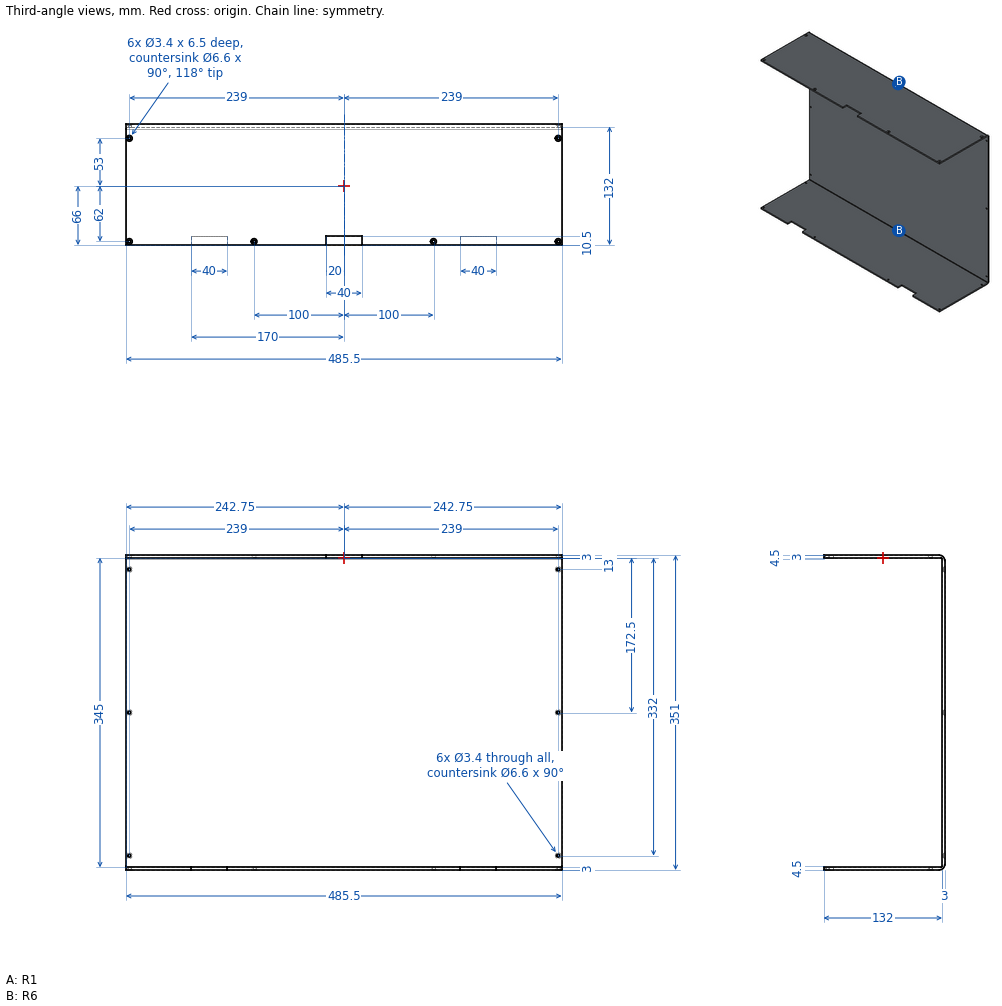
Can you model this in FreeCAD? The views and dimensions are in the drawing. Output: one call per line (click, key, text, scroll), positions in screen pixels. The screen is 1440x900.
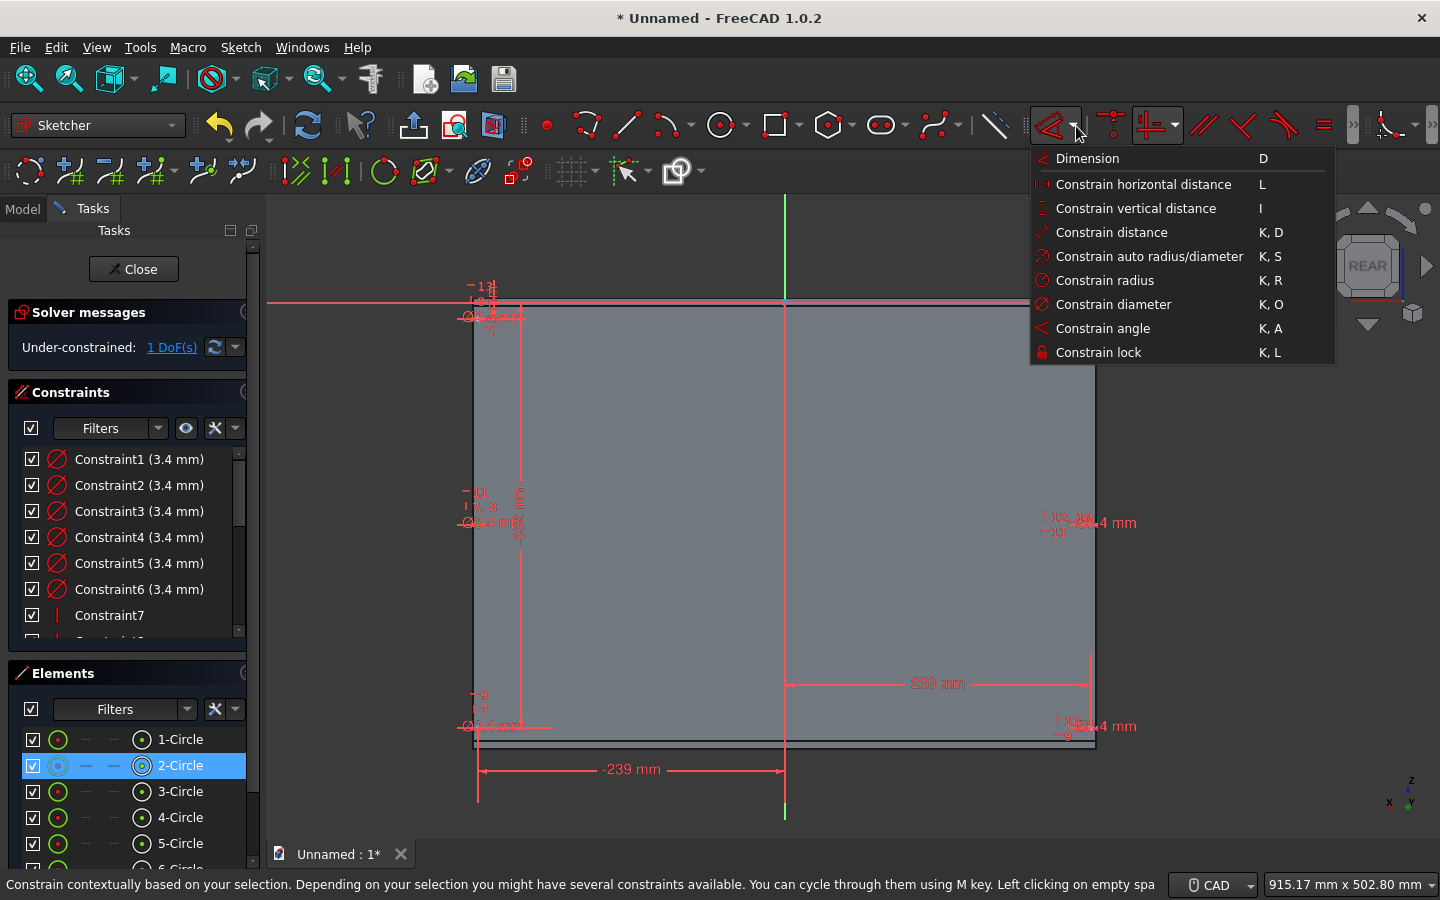
click(1183, 208)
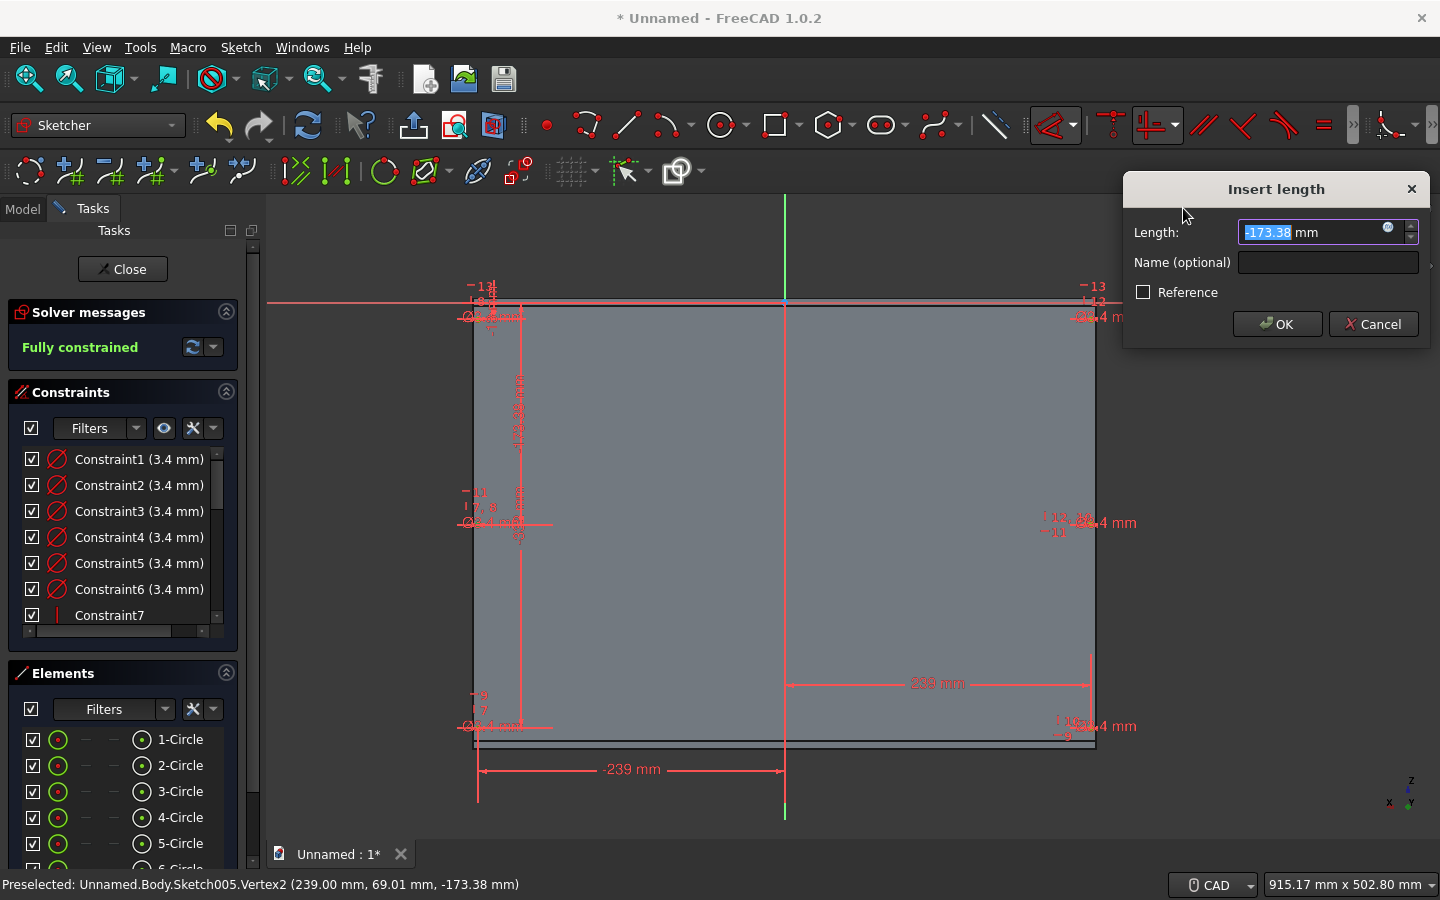
text(-172.5)
key(Return)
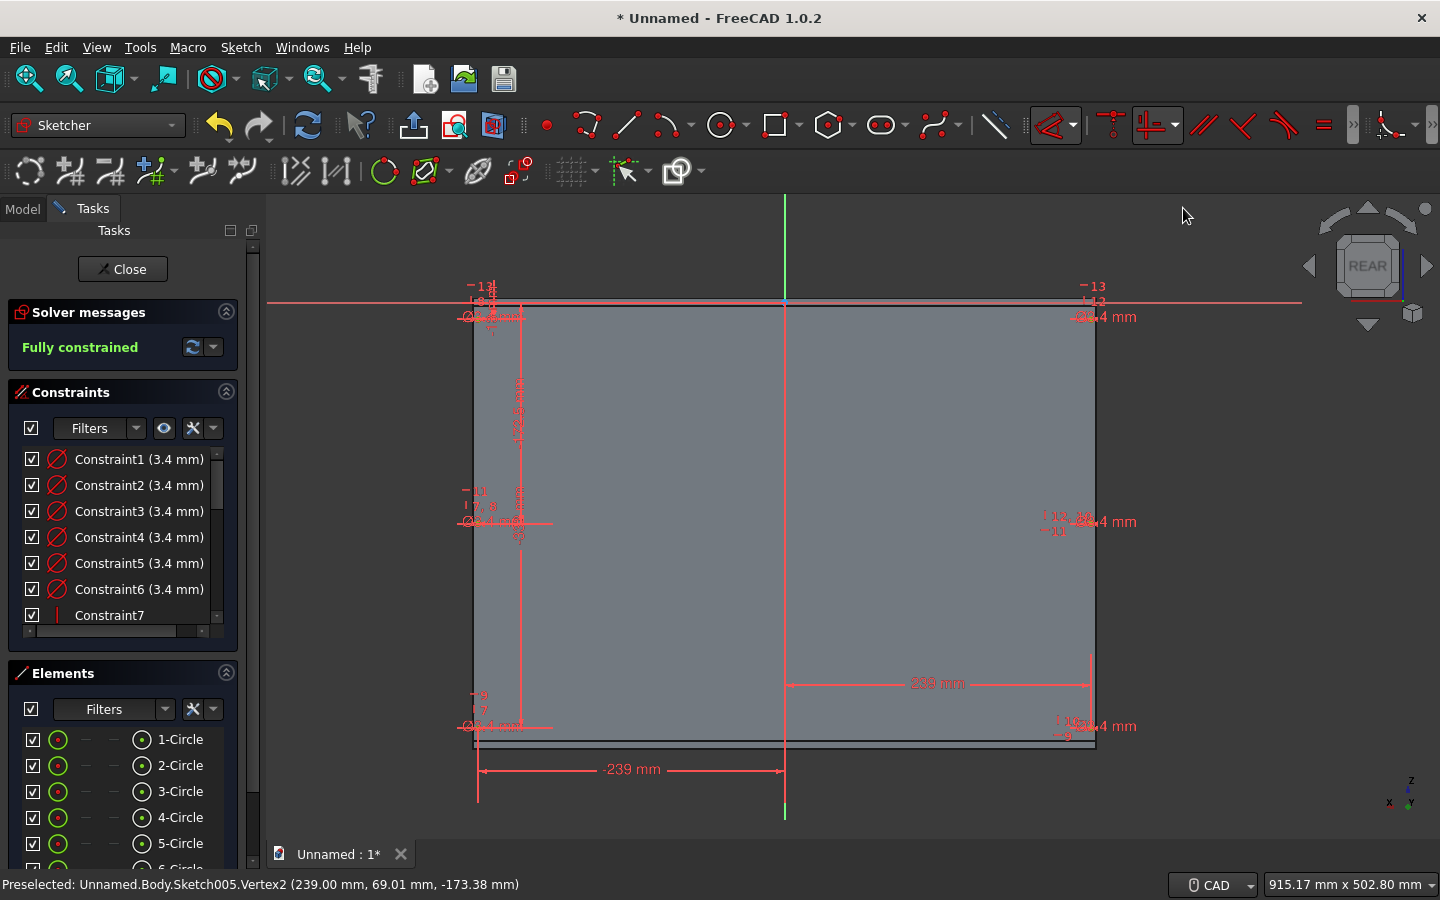
click(123, 269)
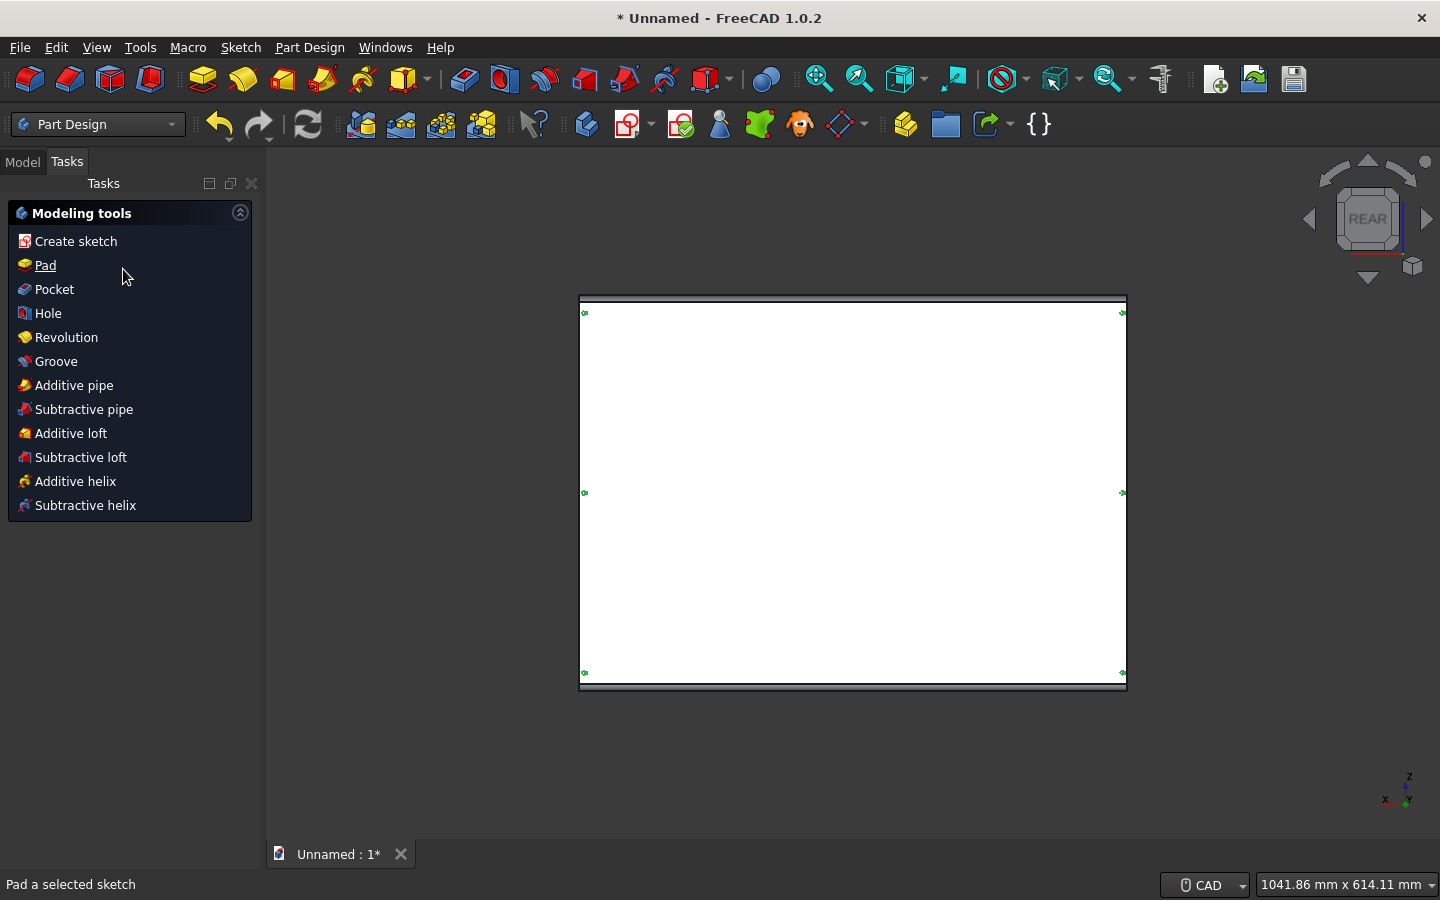
click(506, 80)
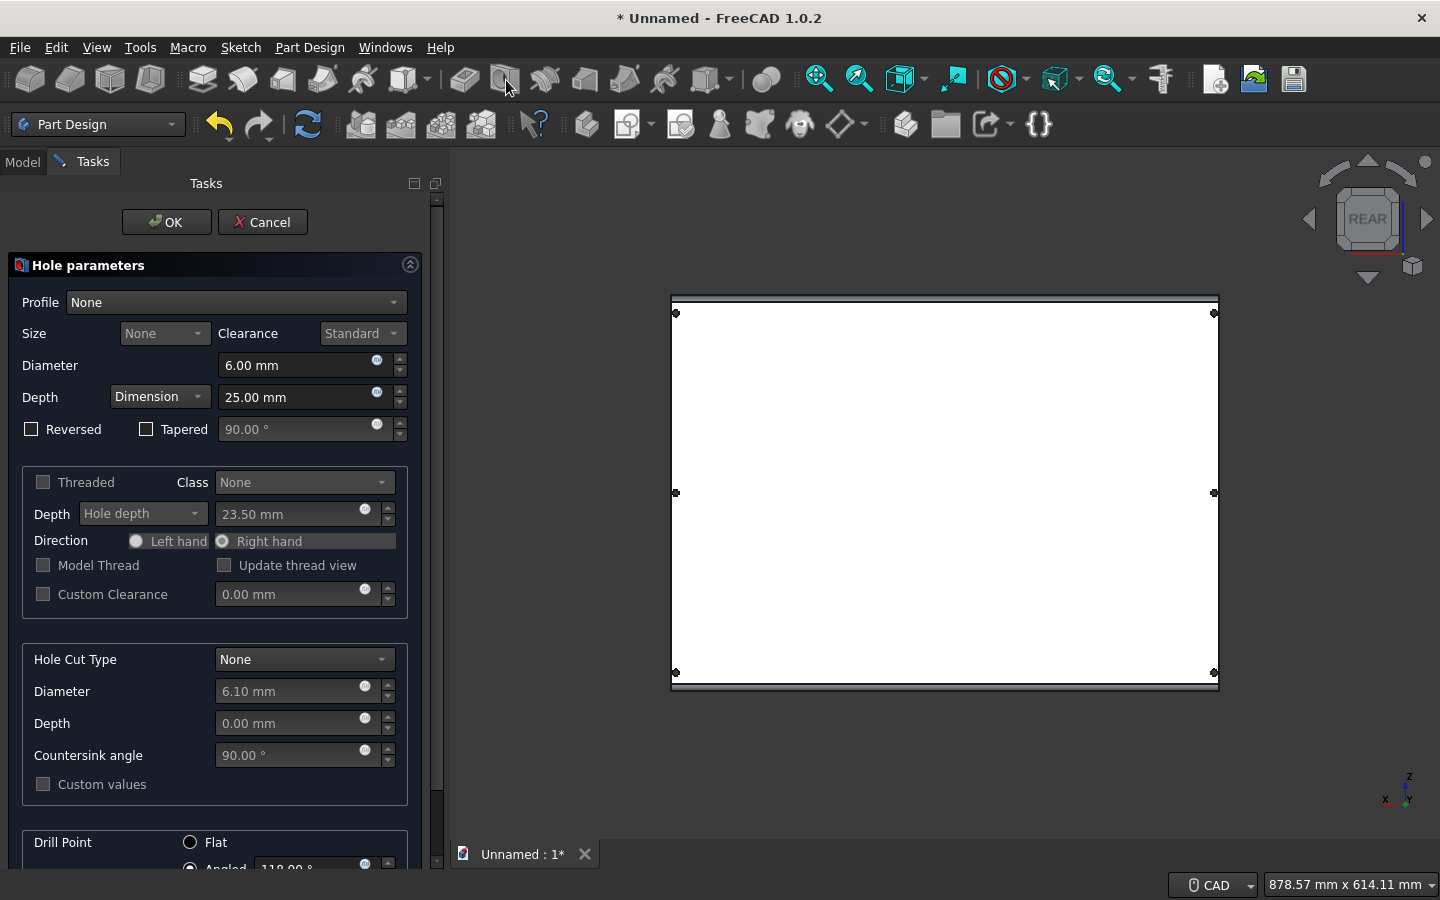
triple_click(305, 365)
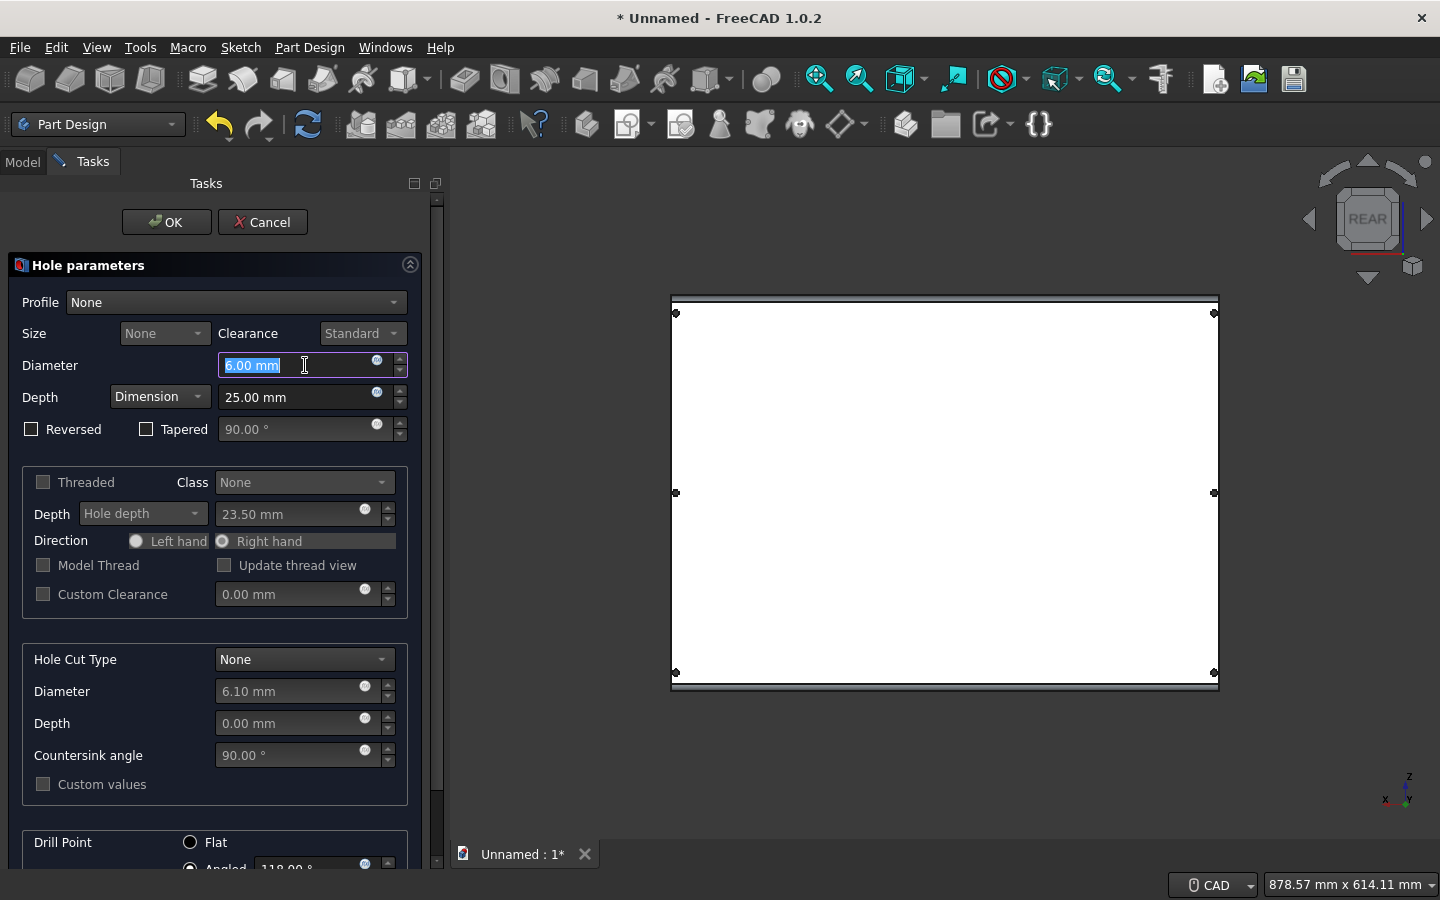
text(3.4)
key(Tab)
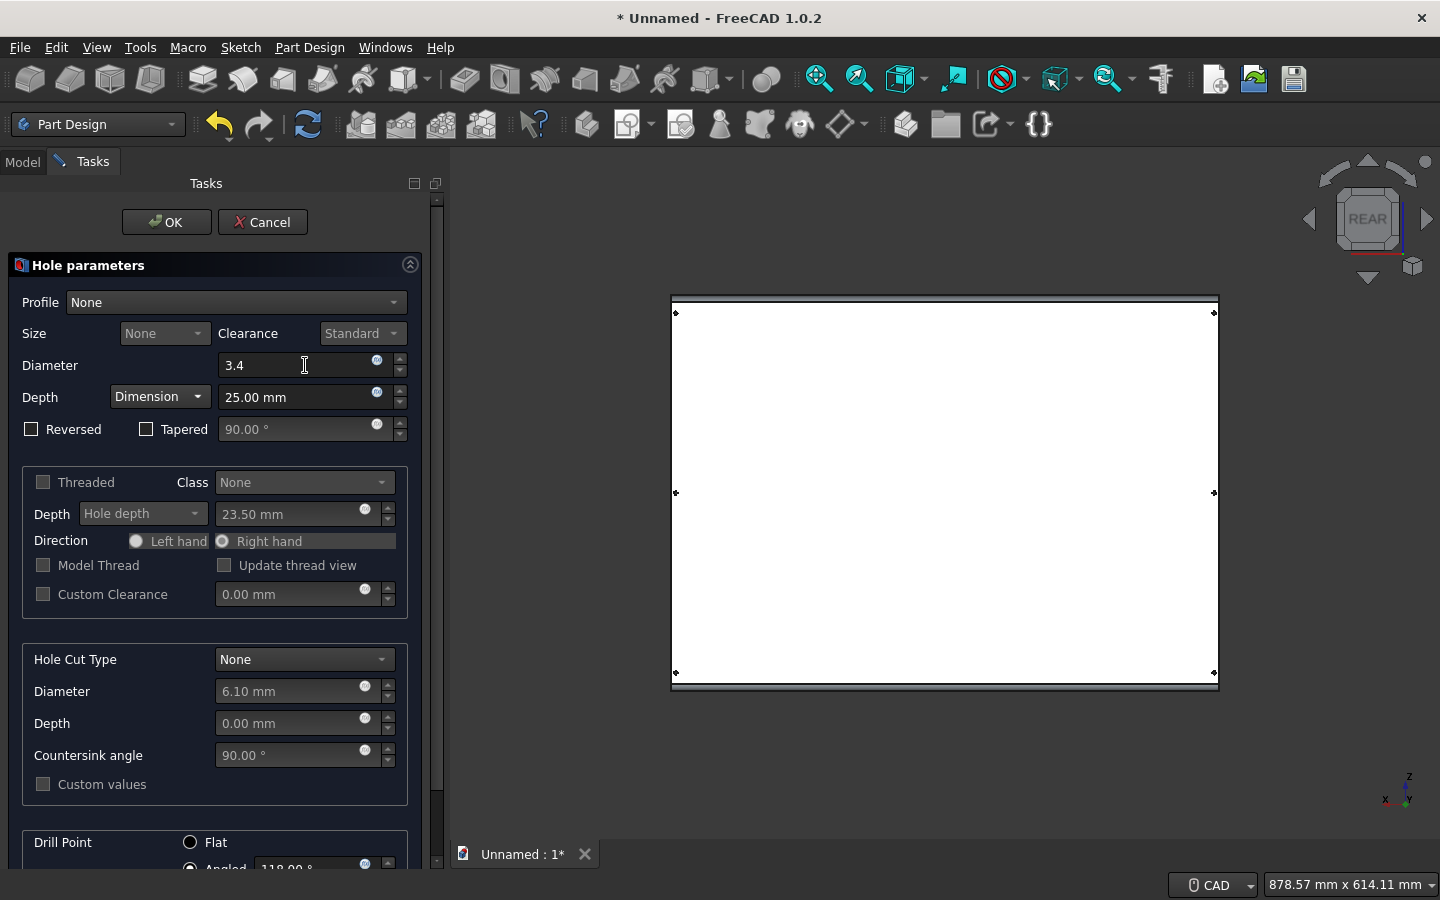
click(161, 396)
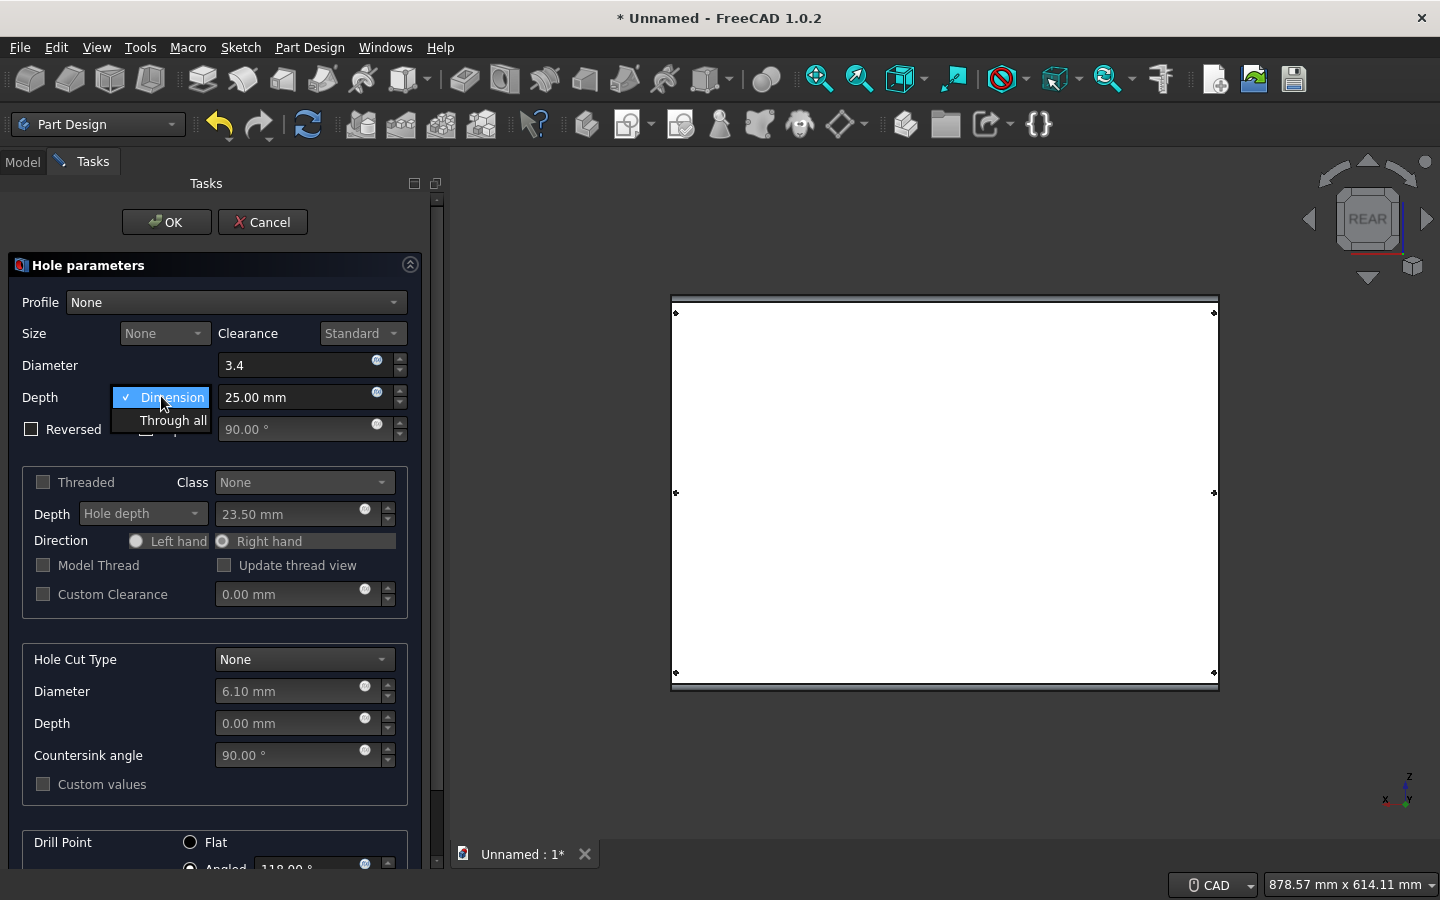
click(160, 420)